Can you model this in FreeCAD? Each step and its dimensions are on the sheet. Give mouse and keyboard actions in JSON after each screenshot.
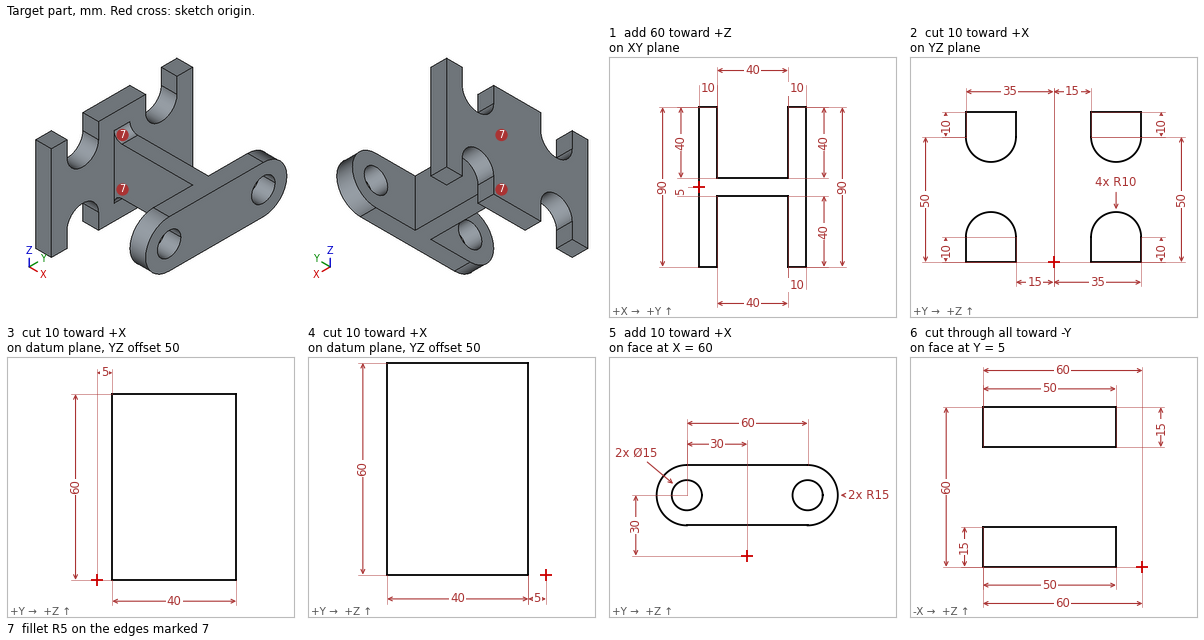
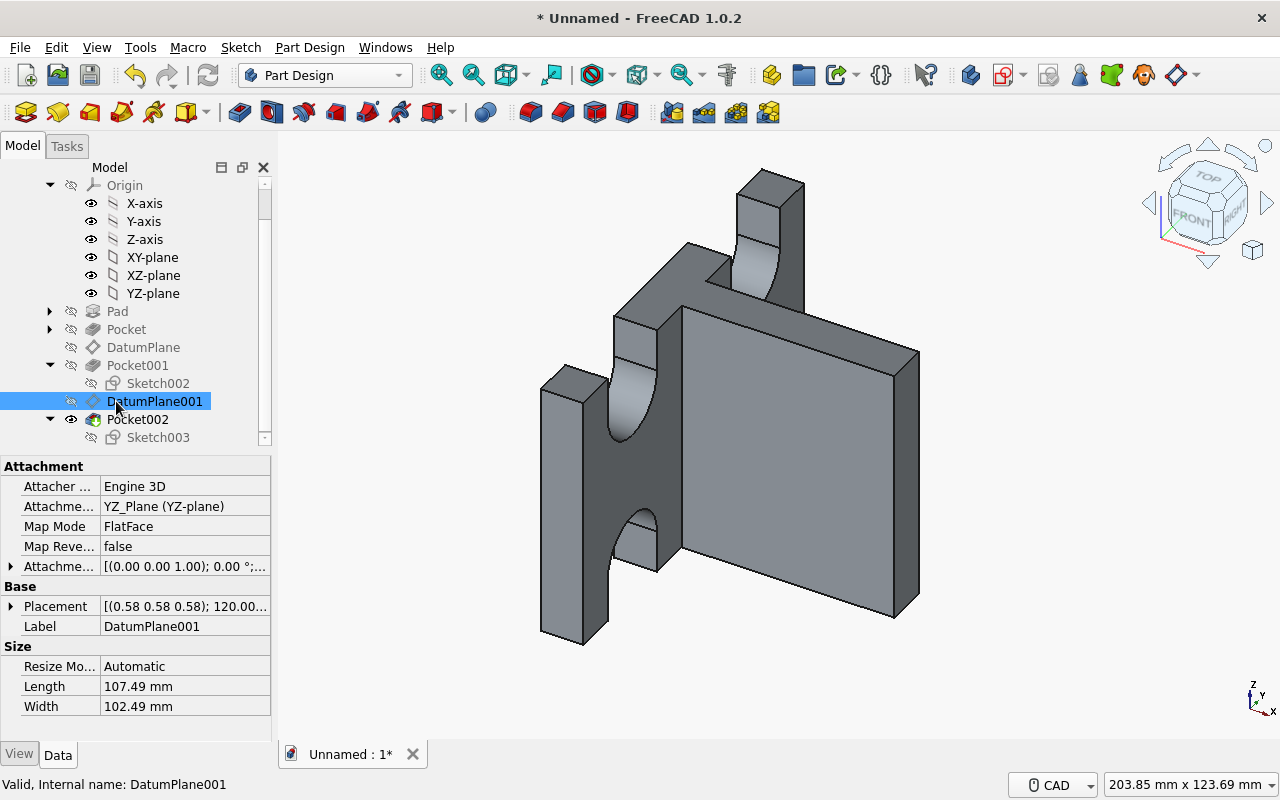
{"action": "left_click", "coordinate": [907, 415]}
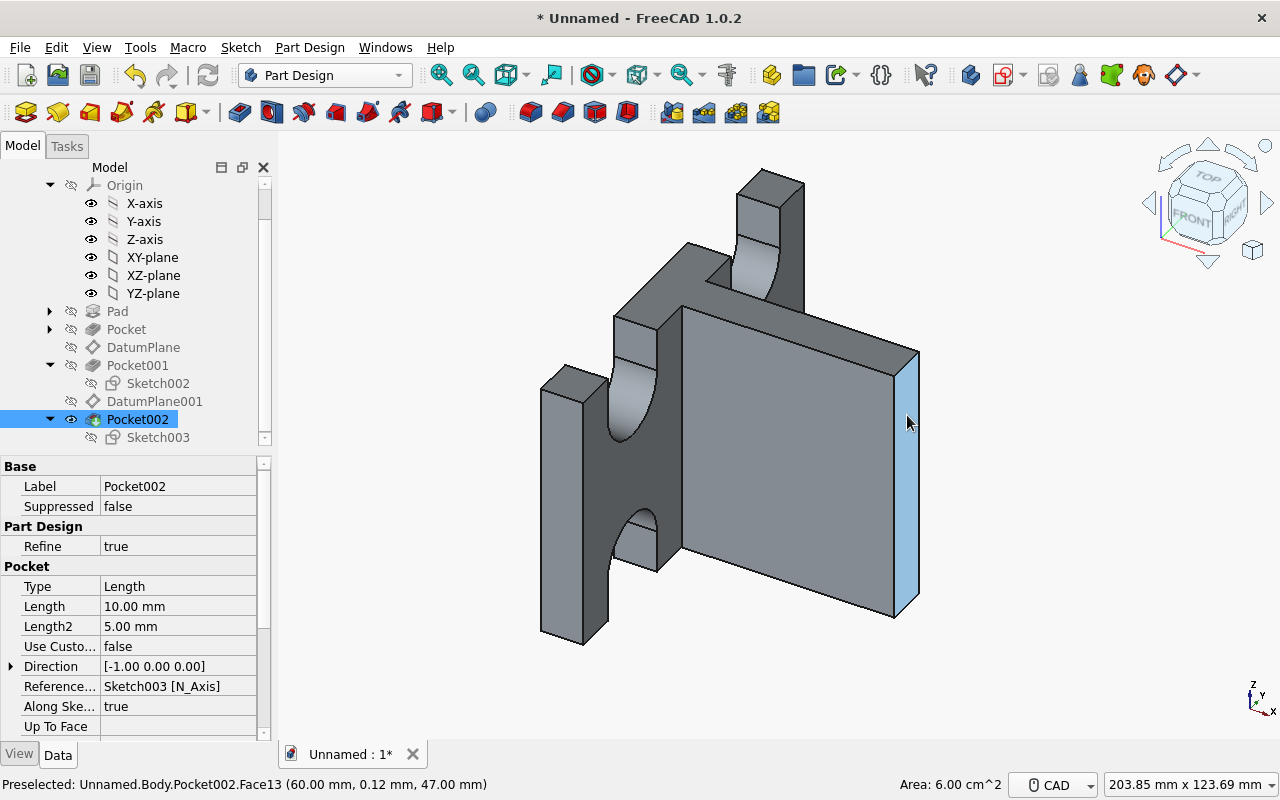
{"action": "left_click", "coordinate": [1004, 76]}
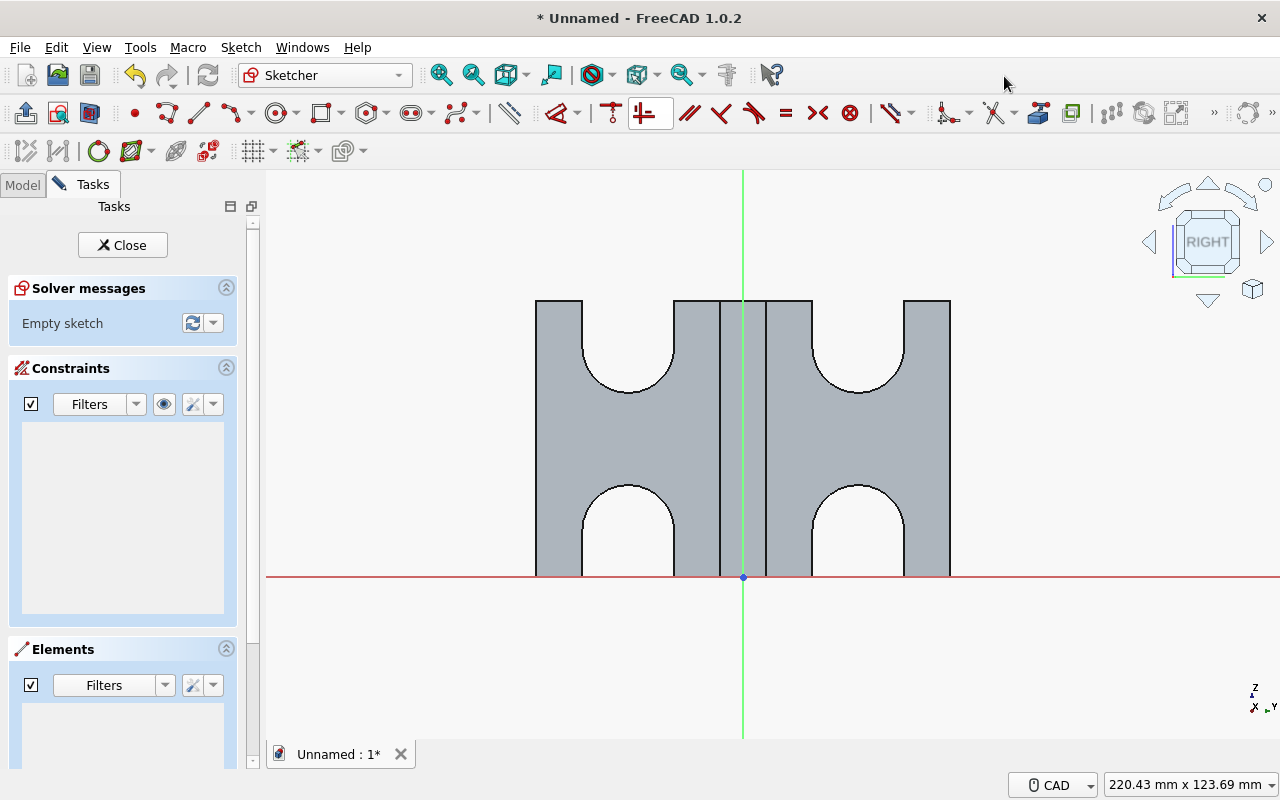
{"action": "scroll", "coordinate": [822, 512], "scroll_direction": "up", "scroll_amount": 2}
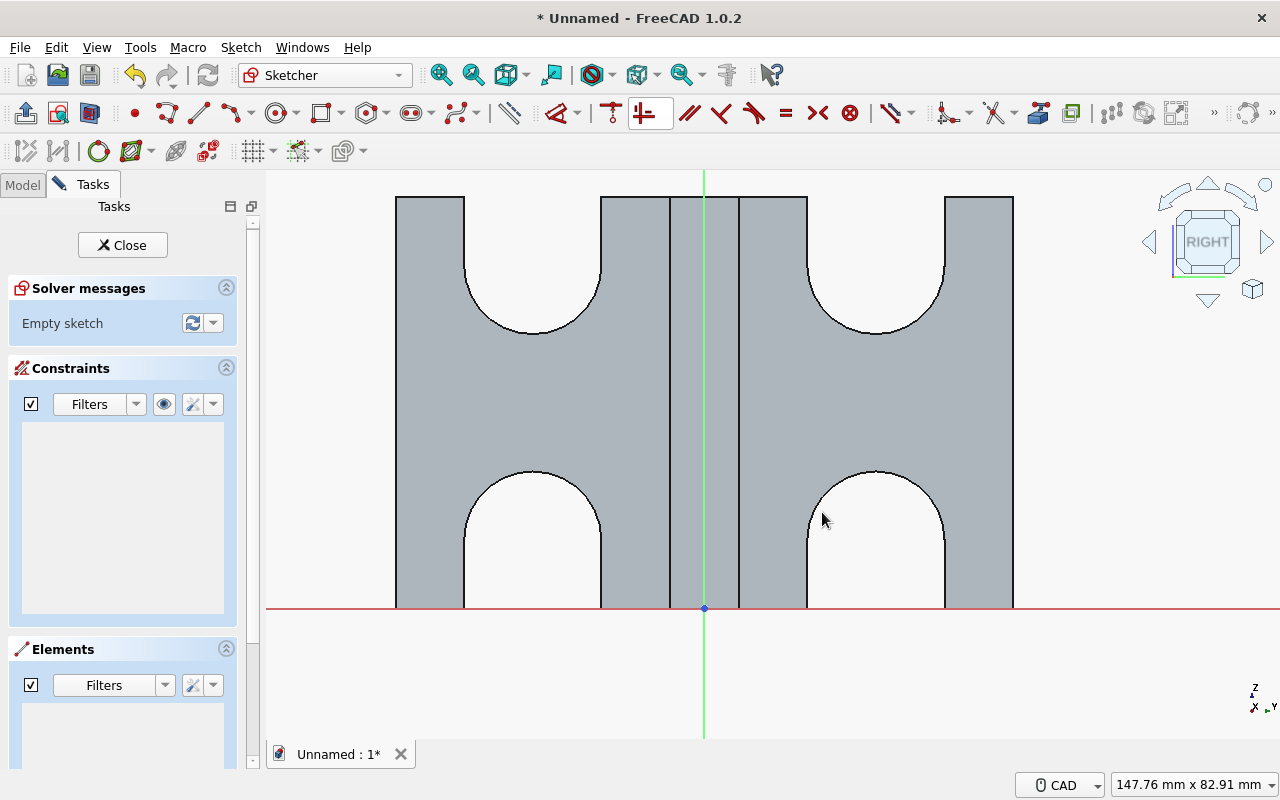
{"action": "left_click", "coordinate": [412, 114]}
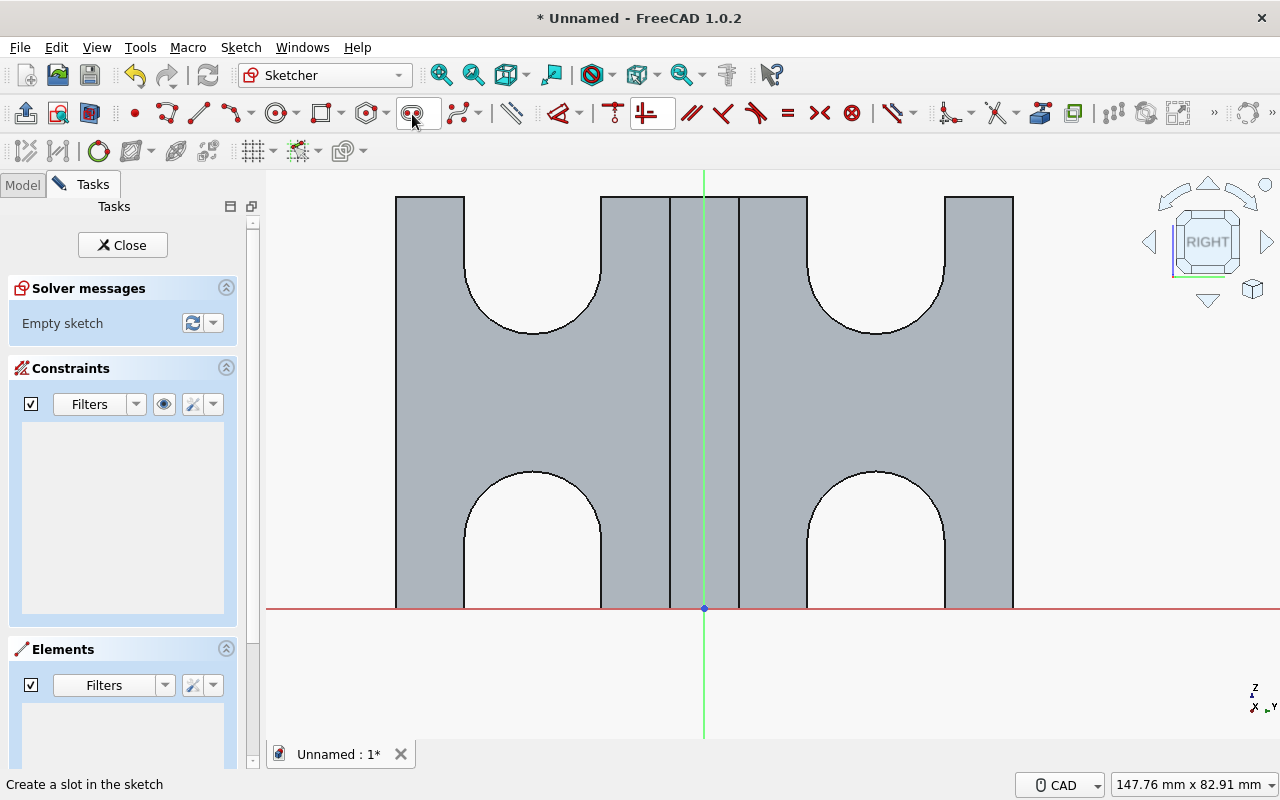
{"action": "left_click", "coordinate": [498, 403]}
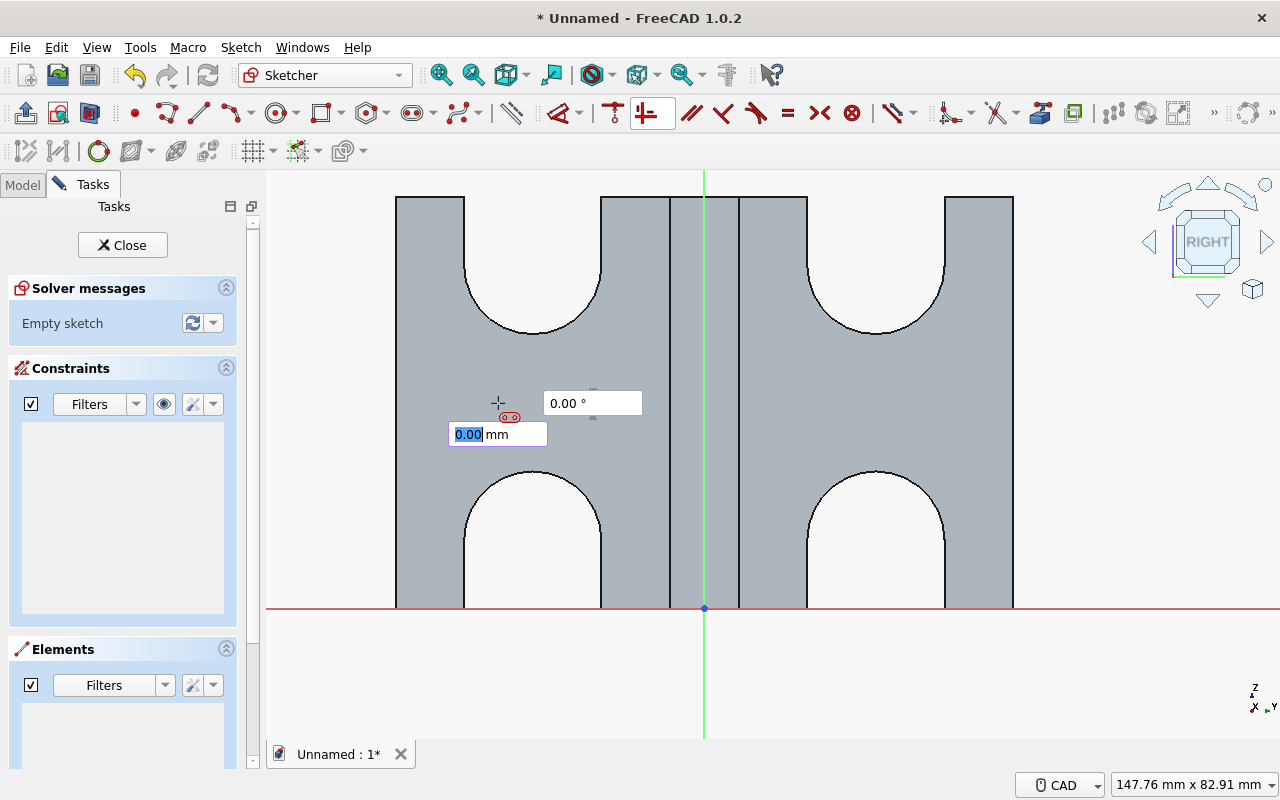
{"action": "left_click", "coordinate": [910, 403]}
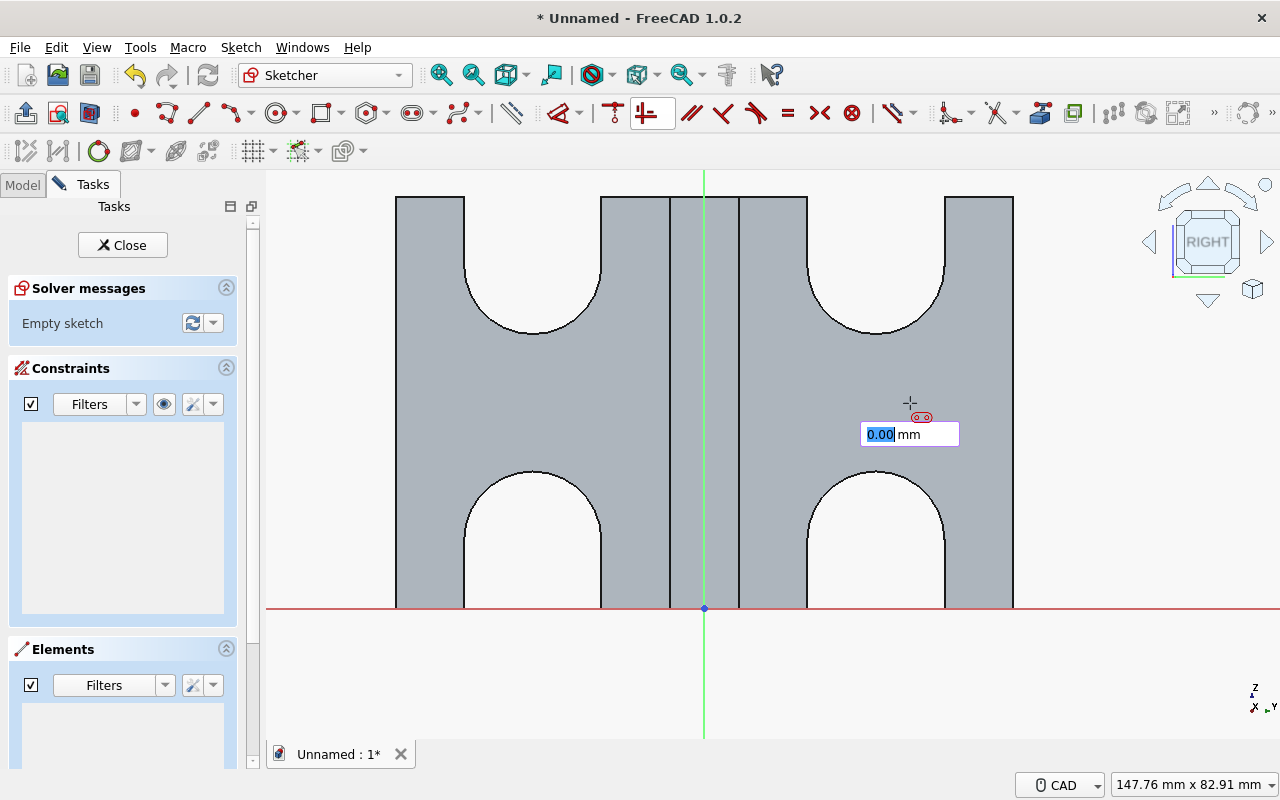
{"action": "left_click", "coordinate": [643, 506]}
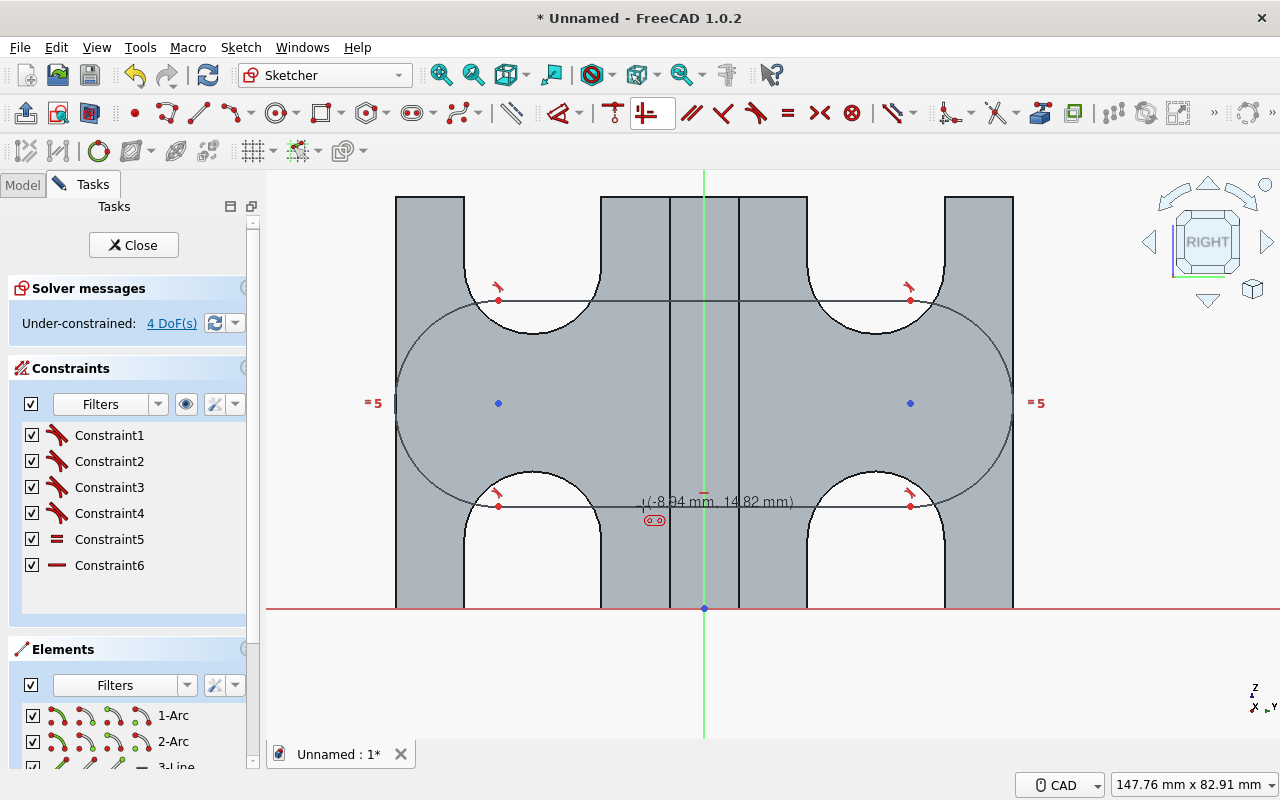
{"action": "left_click", "coordinate": [276, 114]}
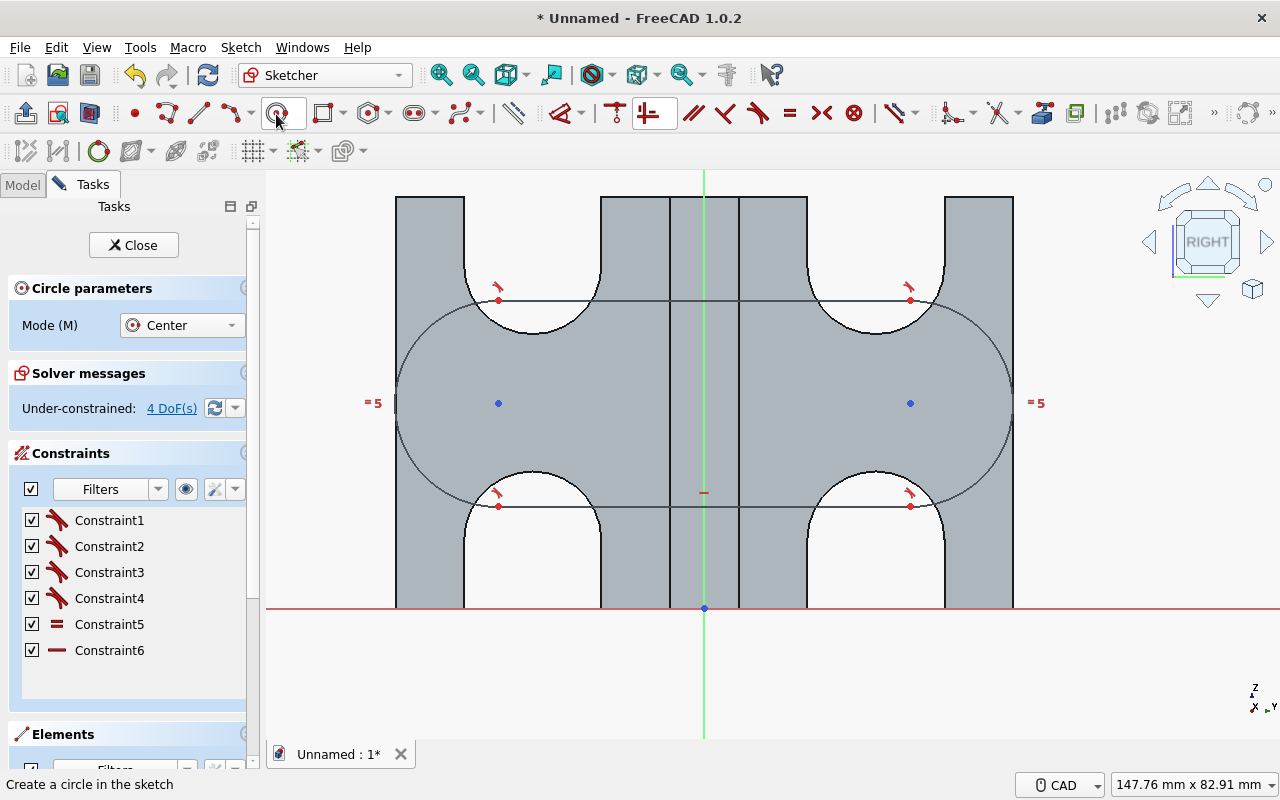
{"action": "left_click", "coordinate": [498, 404]}
{"action": "mouse_move", "coordinate": [535, 366]}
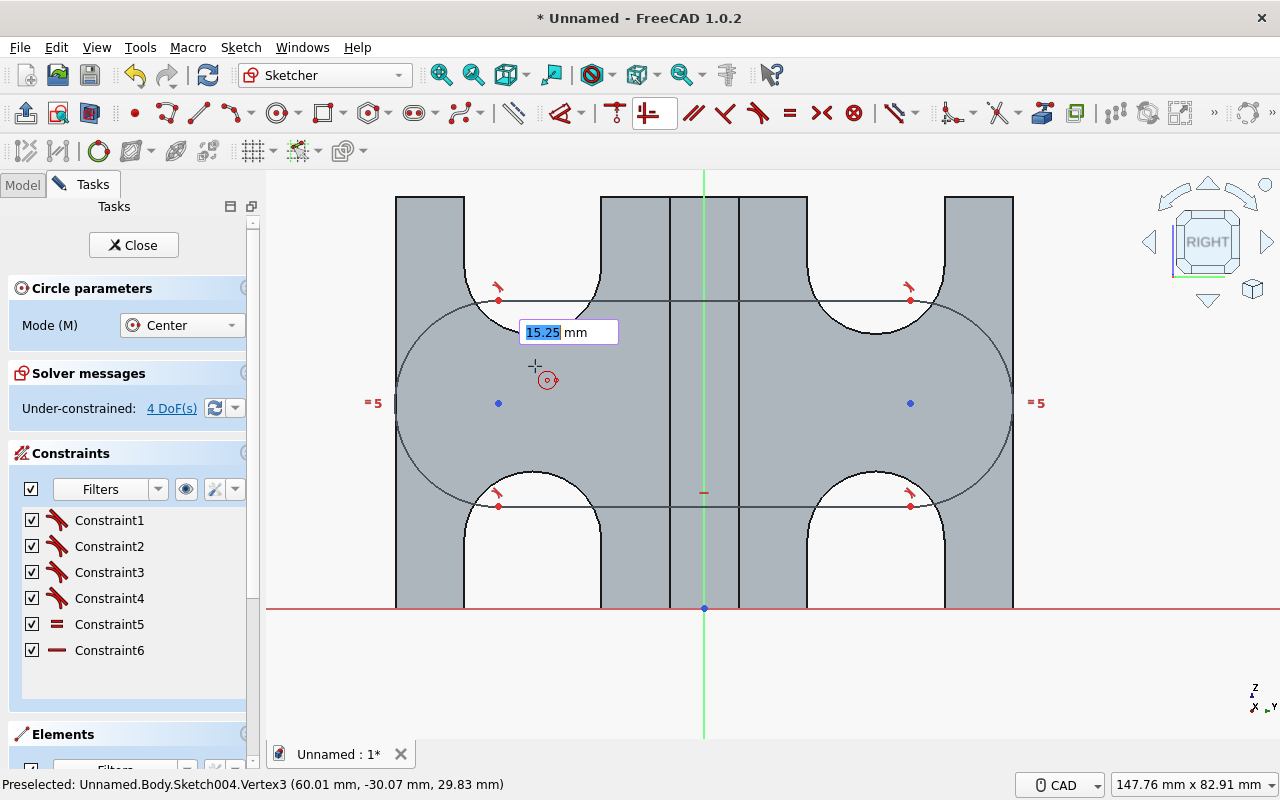
{"action": "type", "text": "15"}
{"action": "key", "text": "Return"}